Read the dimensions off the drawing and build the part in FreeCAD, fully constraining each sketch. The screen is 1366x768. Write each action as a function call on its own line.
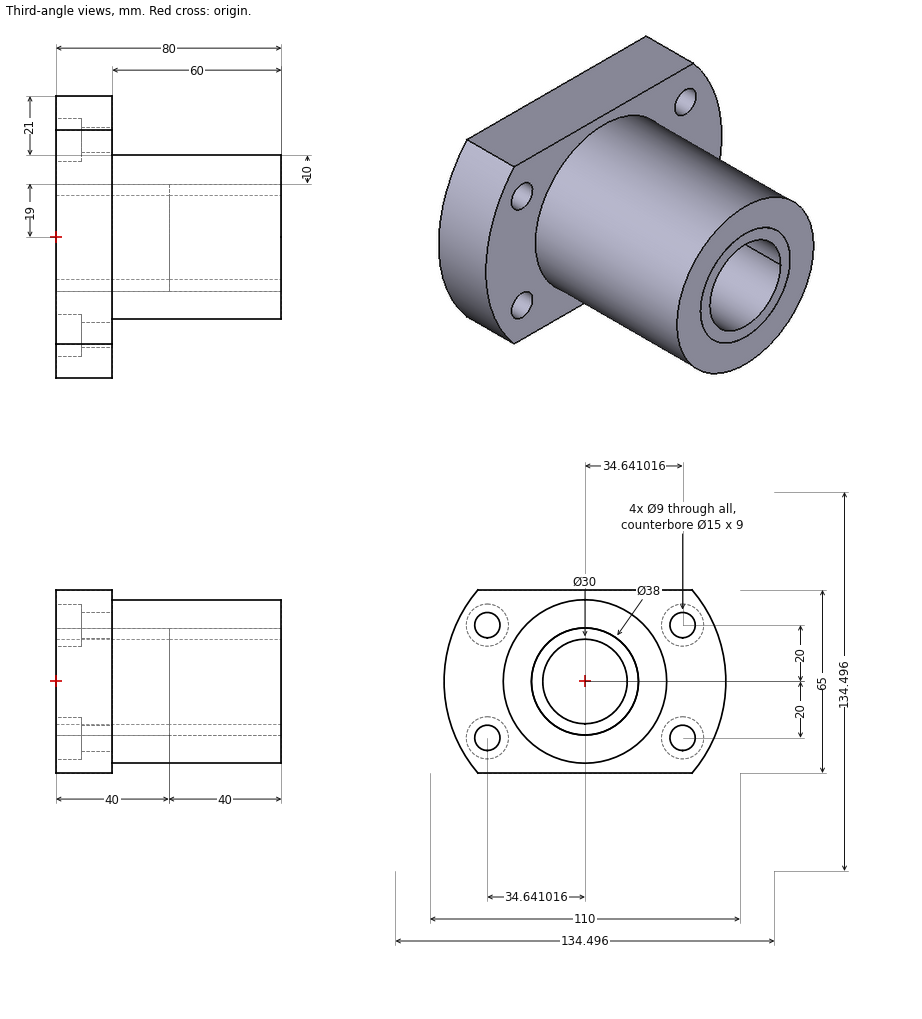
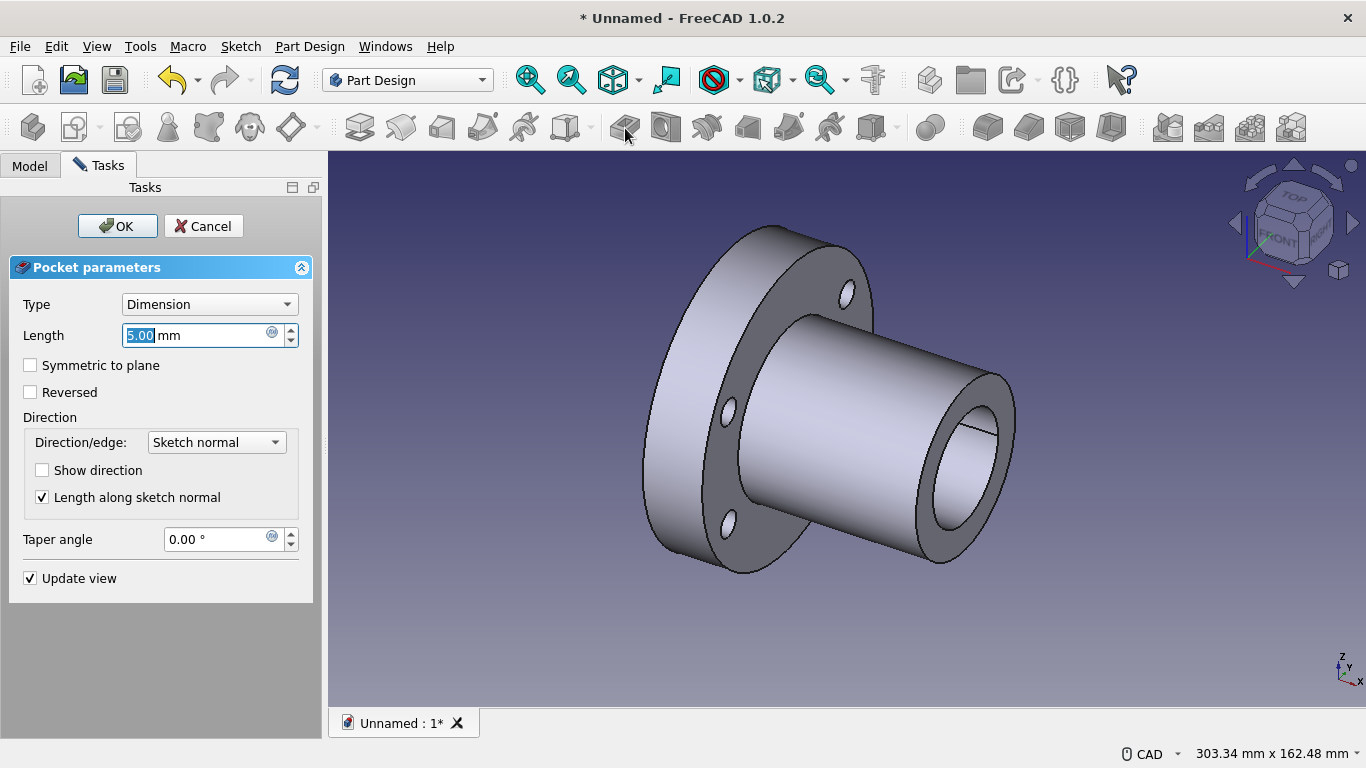
click(210, 304)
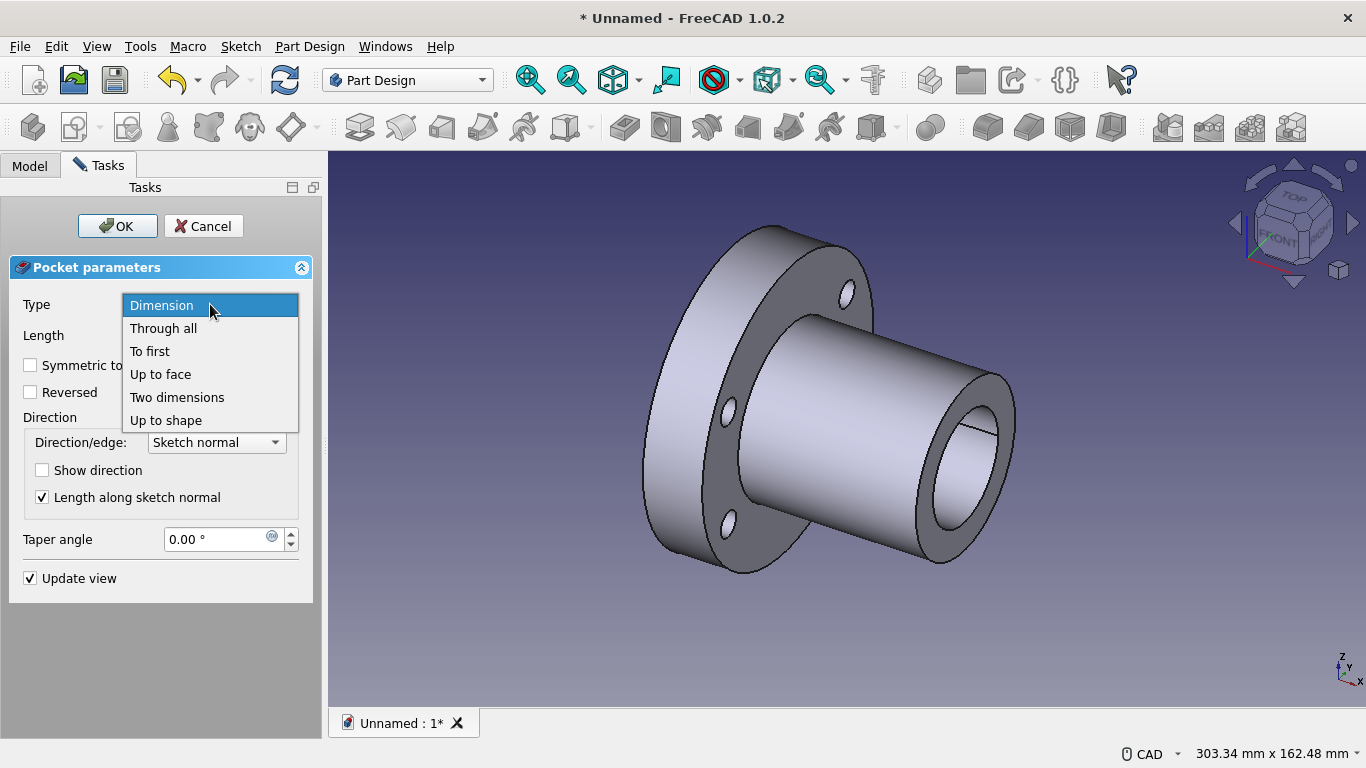
click(208, 328)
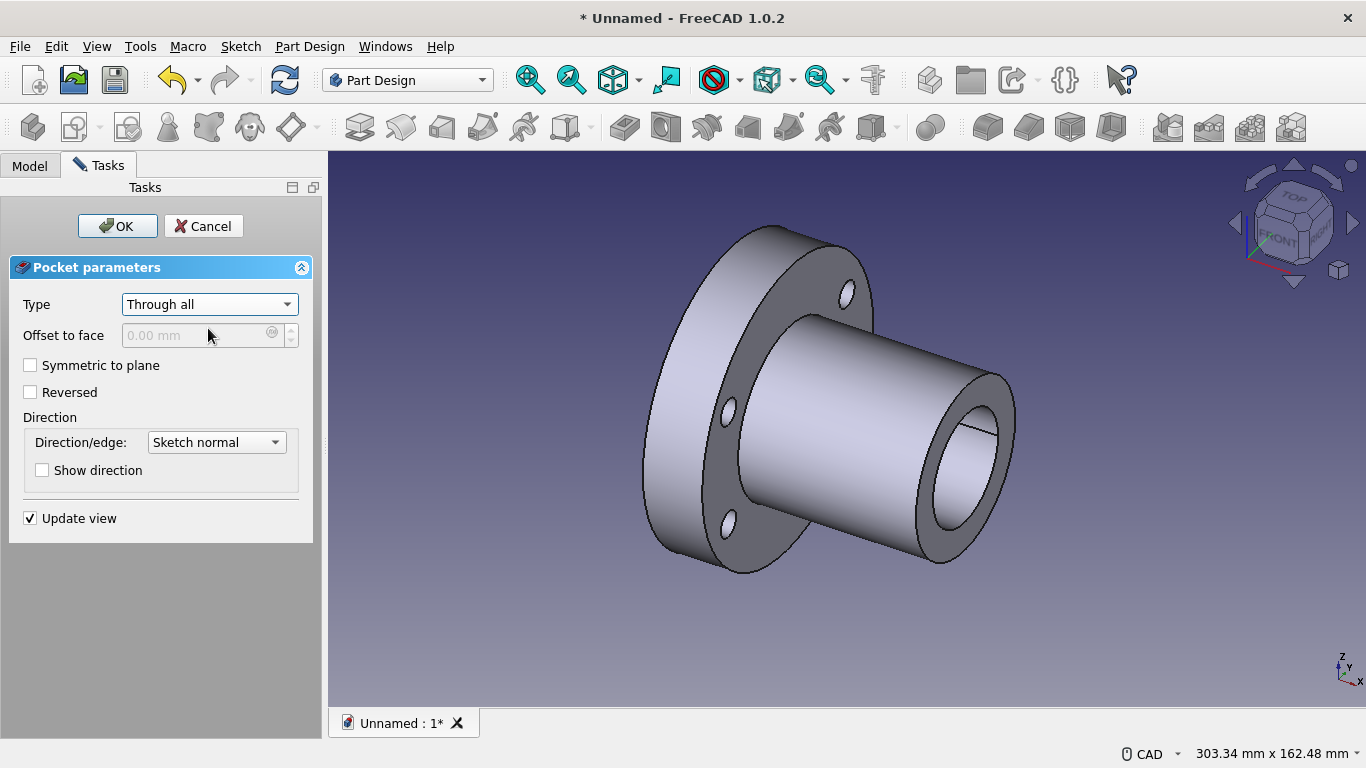
click(31, 392)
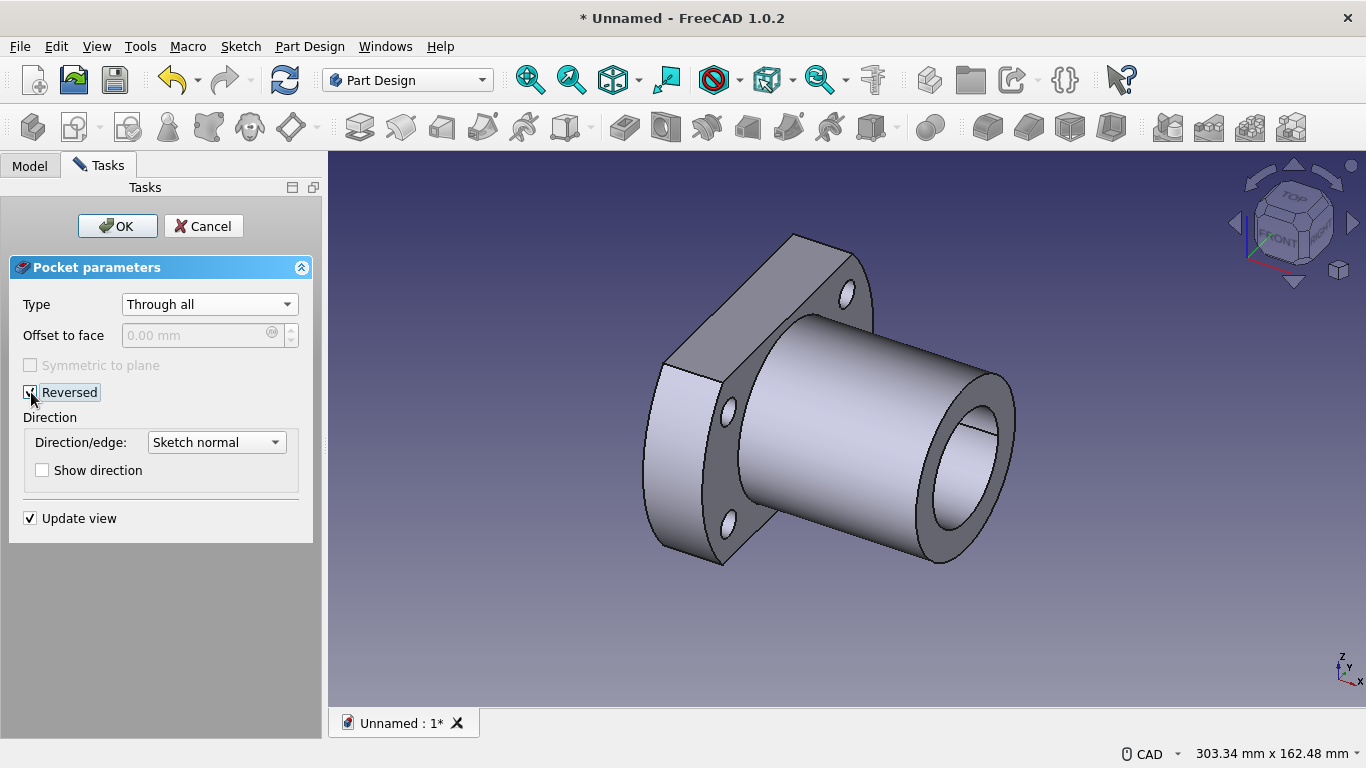
click(118, 226)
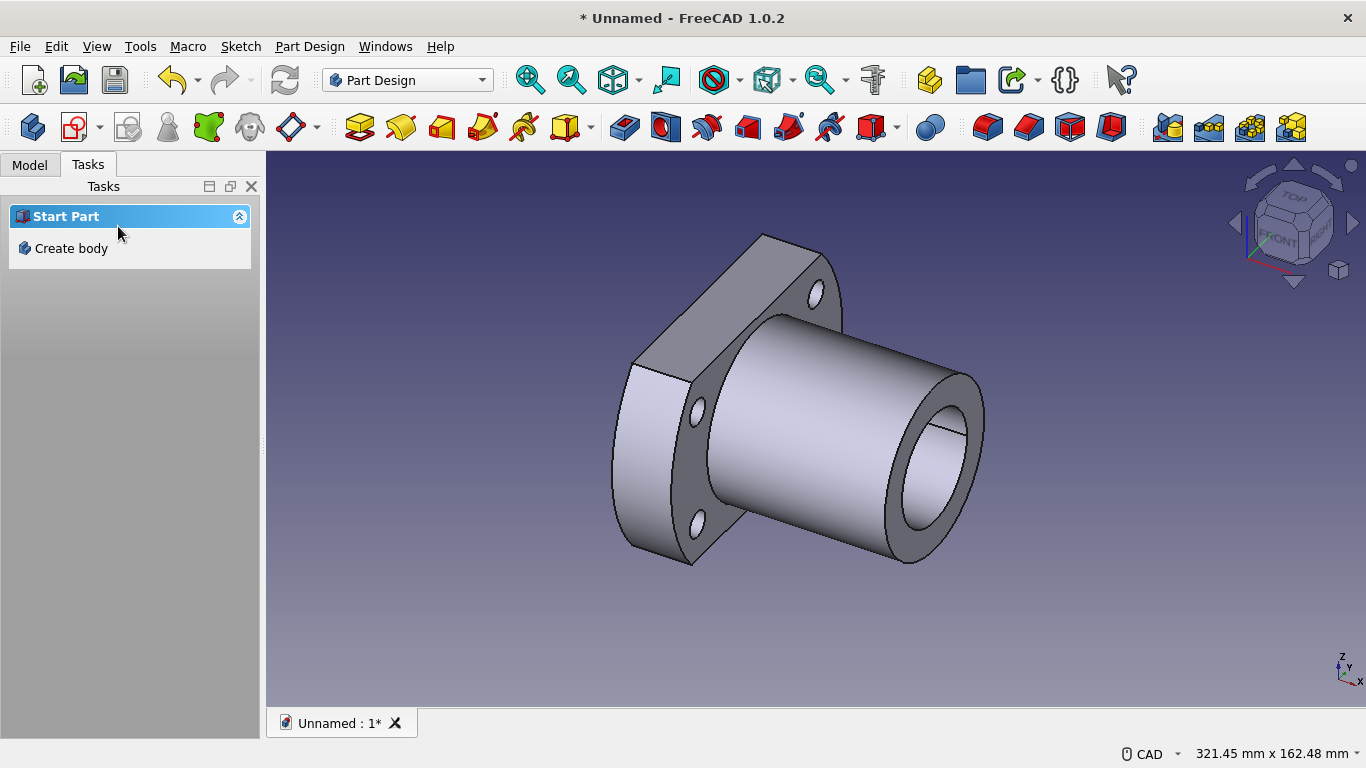
click(33, 128)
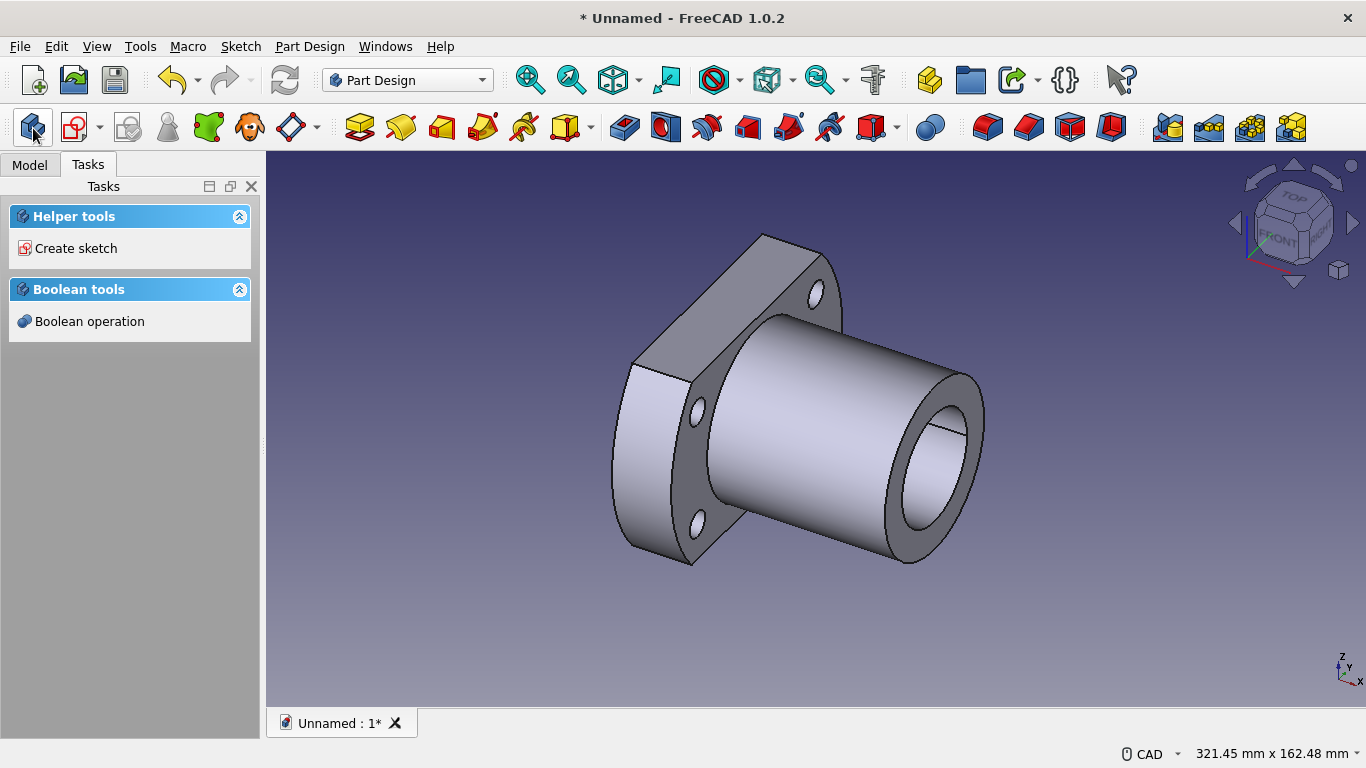
click(30, 164)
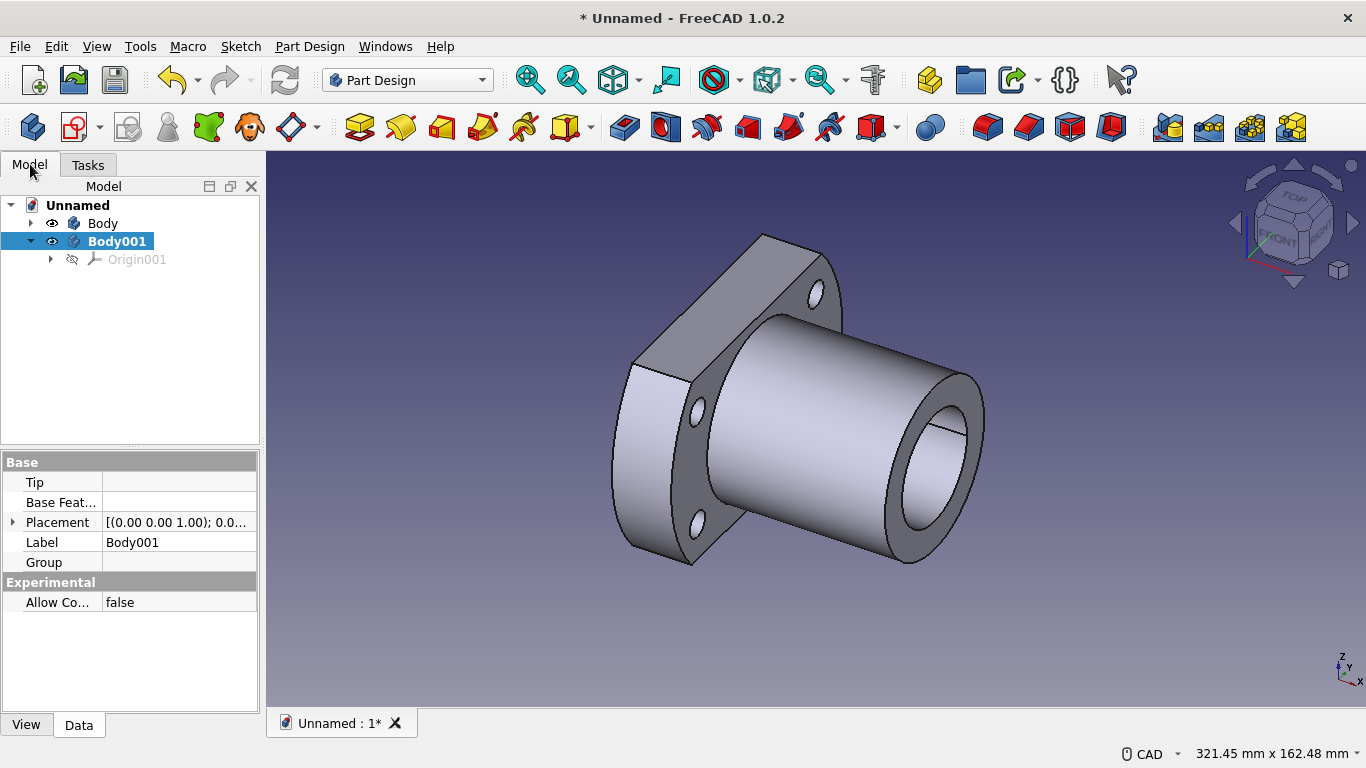
click(51, 259)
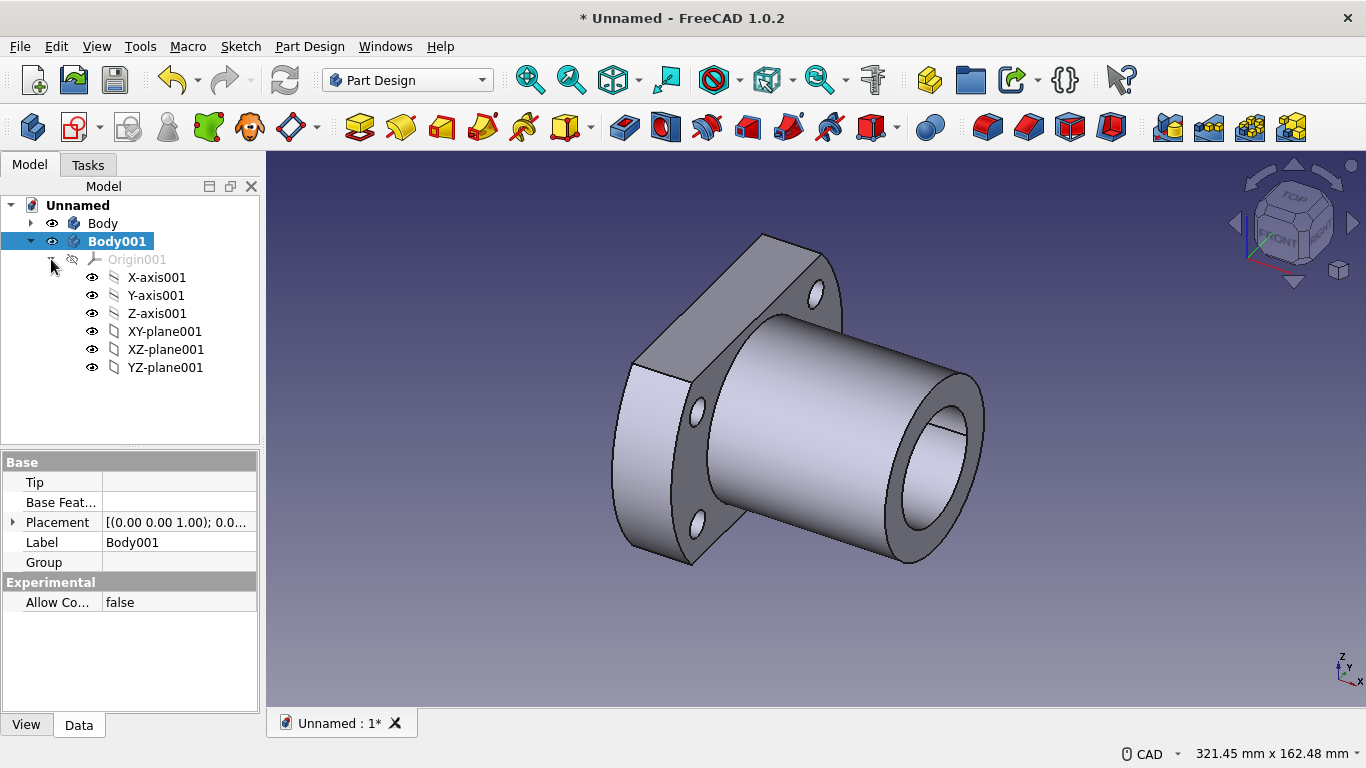
click(137, 367)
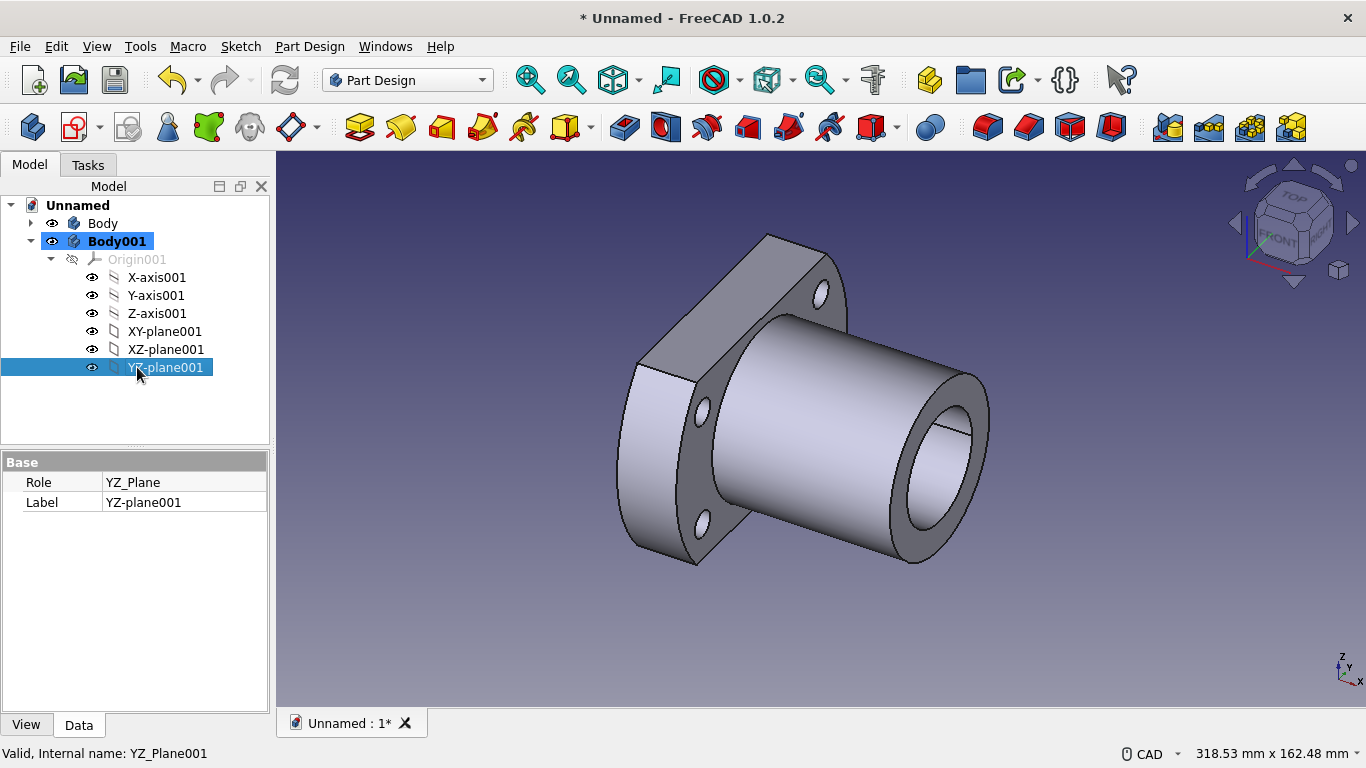
click(290, 128)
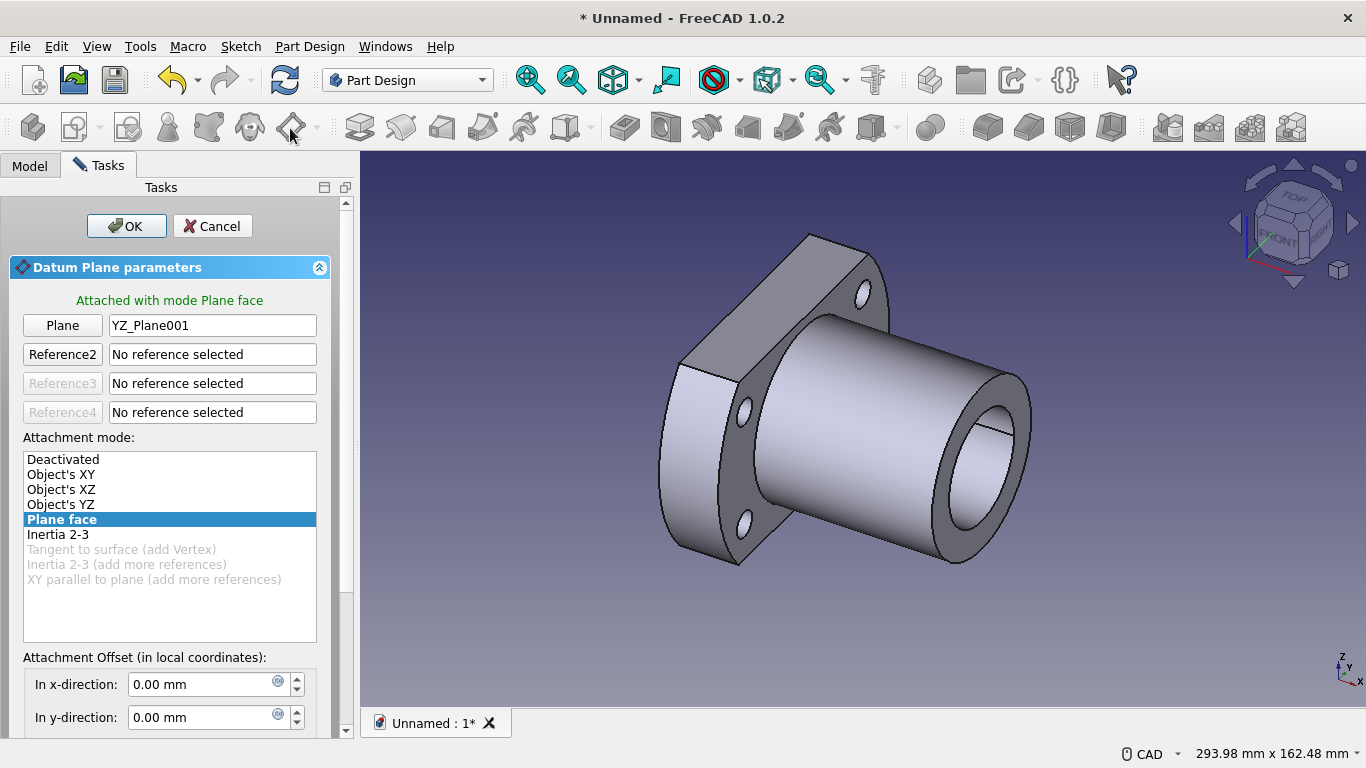
scroll(346, 468, down, 2)